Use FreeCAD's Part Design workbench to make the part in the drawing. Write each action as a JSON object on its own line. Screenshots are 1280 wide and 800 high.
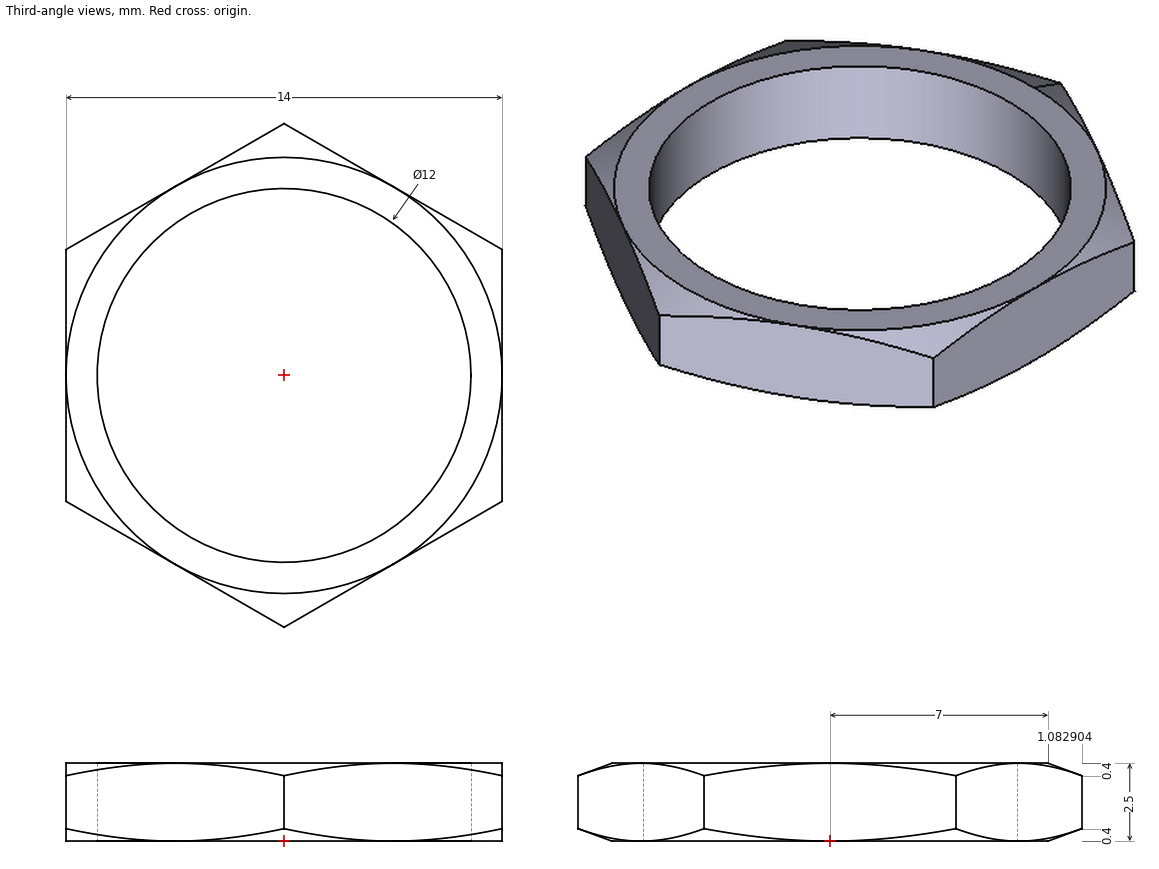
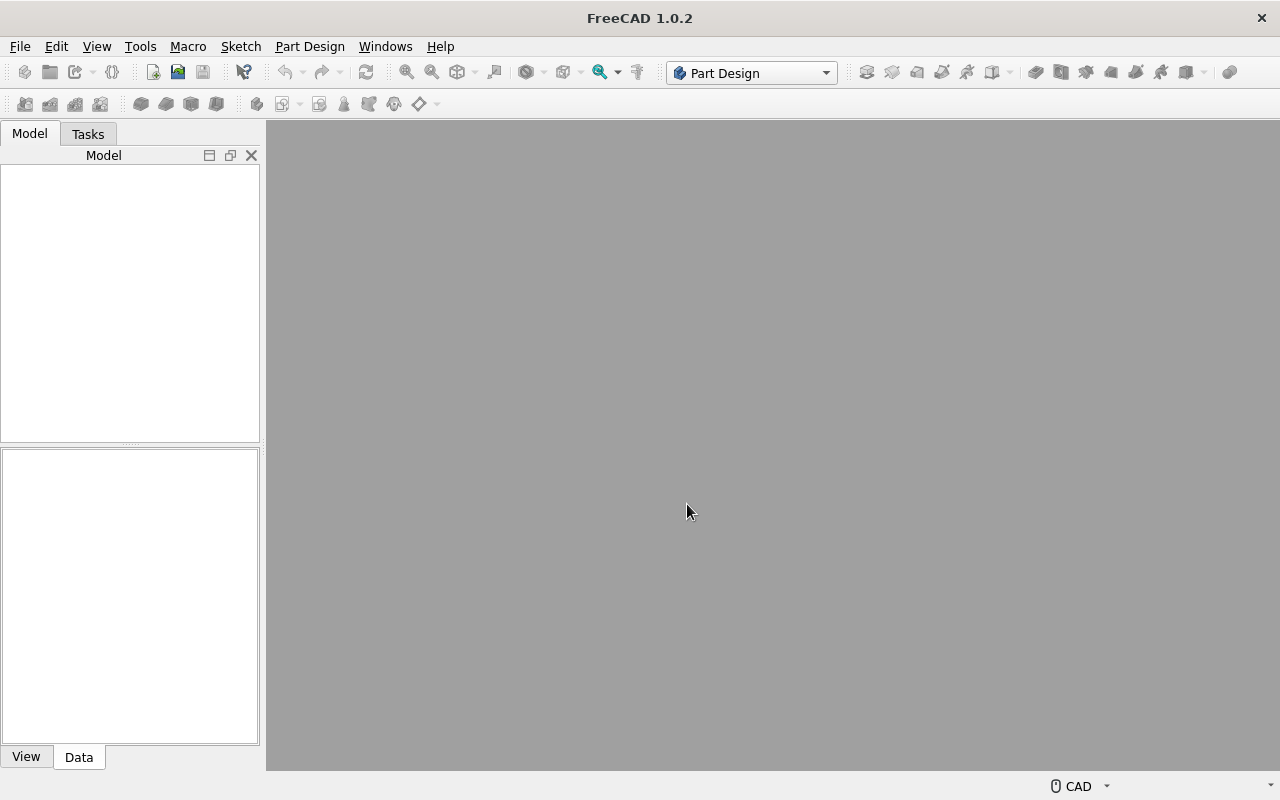
{"action": "key", "text": "ctrl+n"}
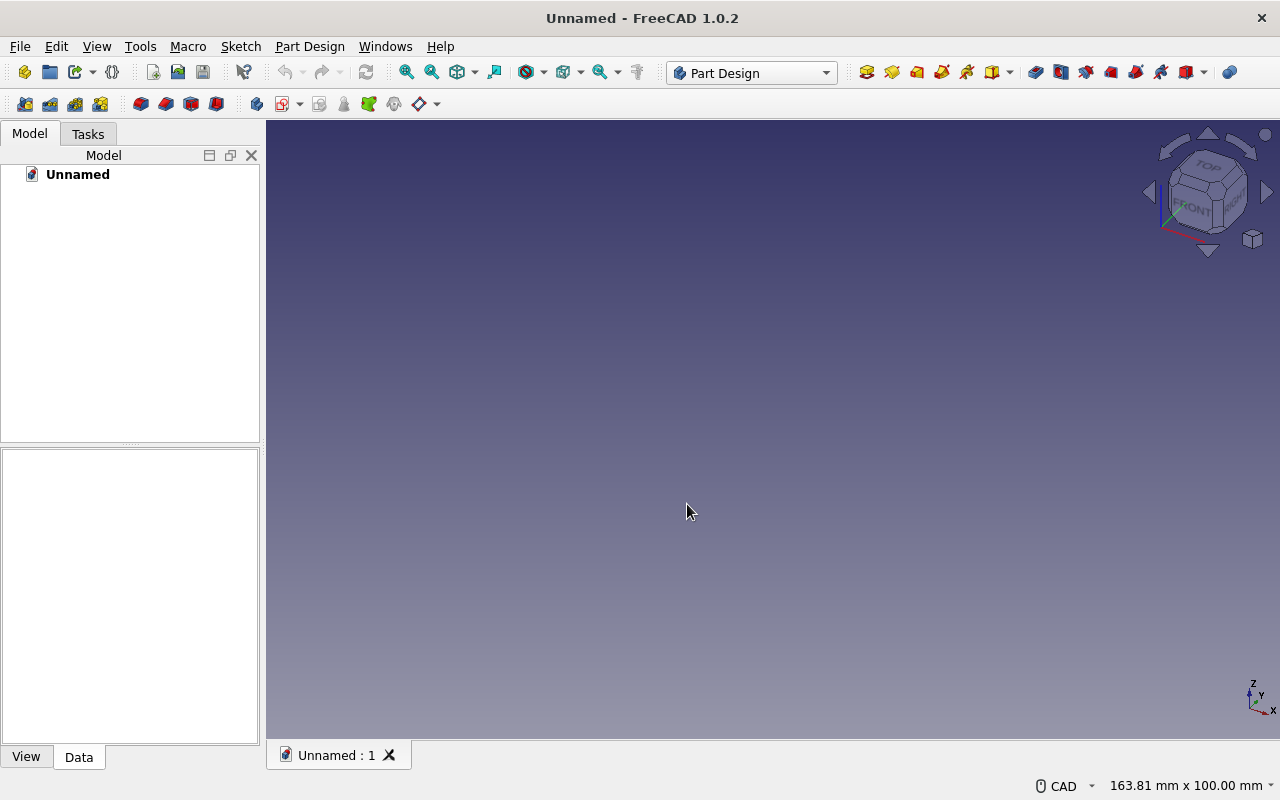
{"action": "left_click", "coordinate": [282, 104]}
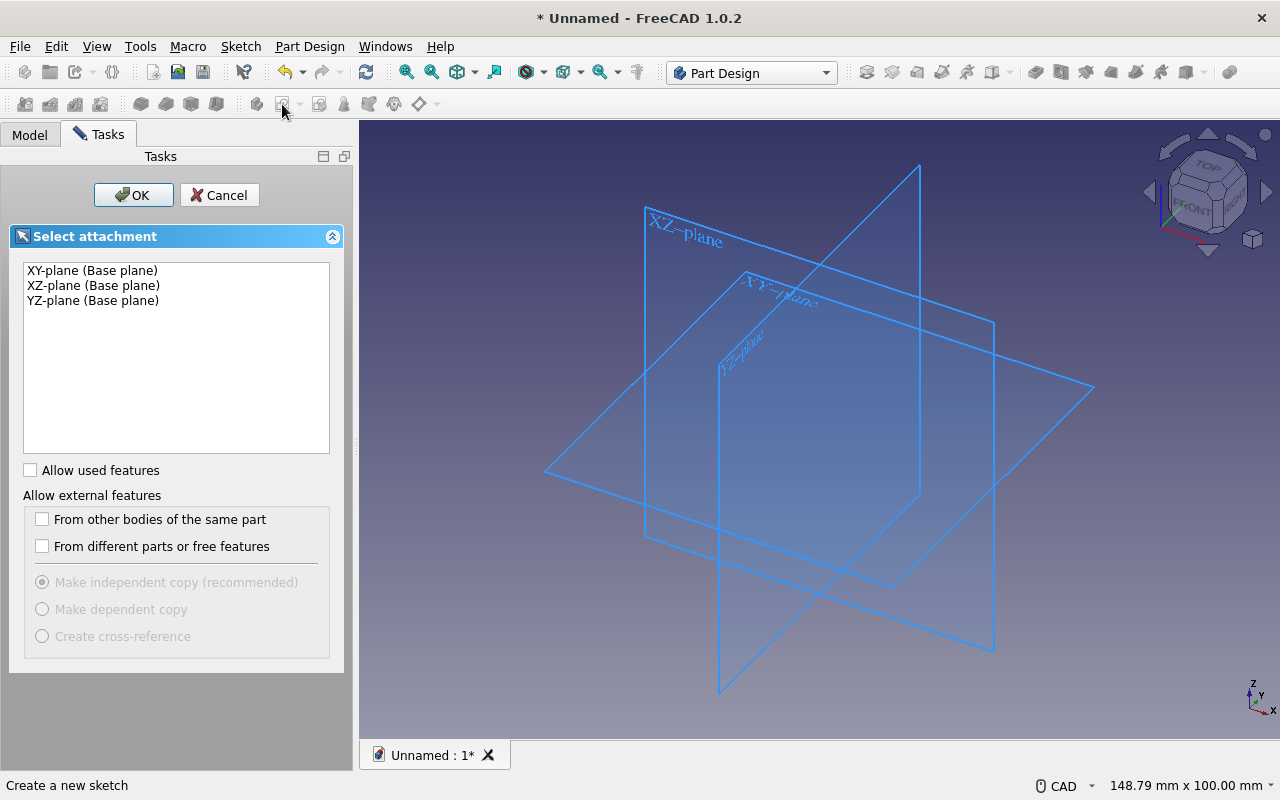
{"action": "left_click", "coordinate": [84, 270]}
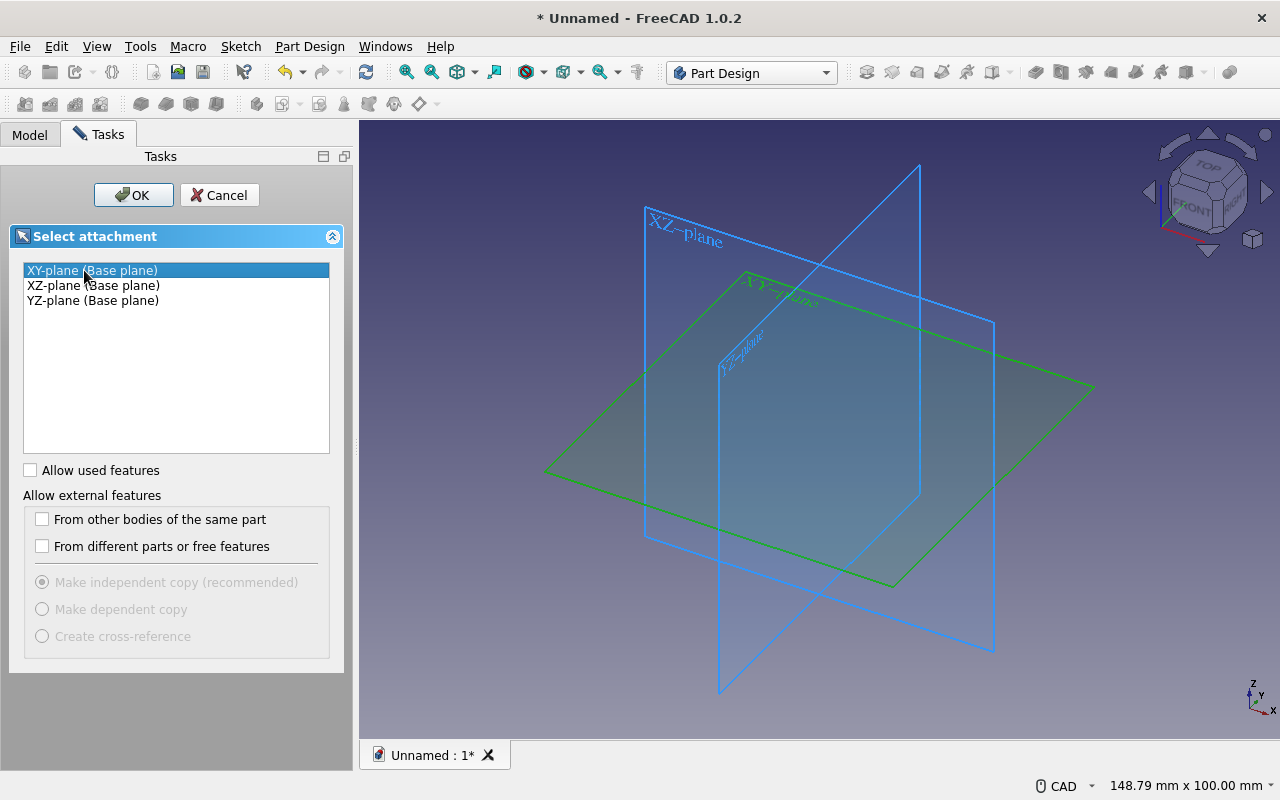
{"action": "left_click", "coordinate": [134, 195]}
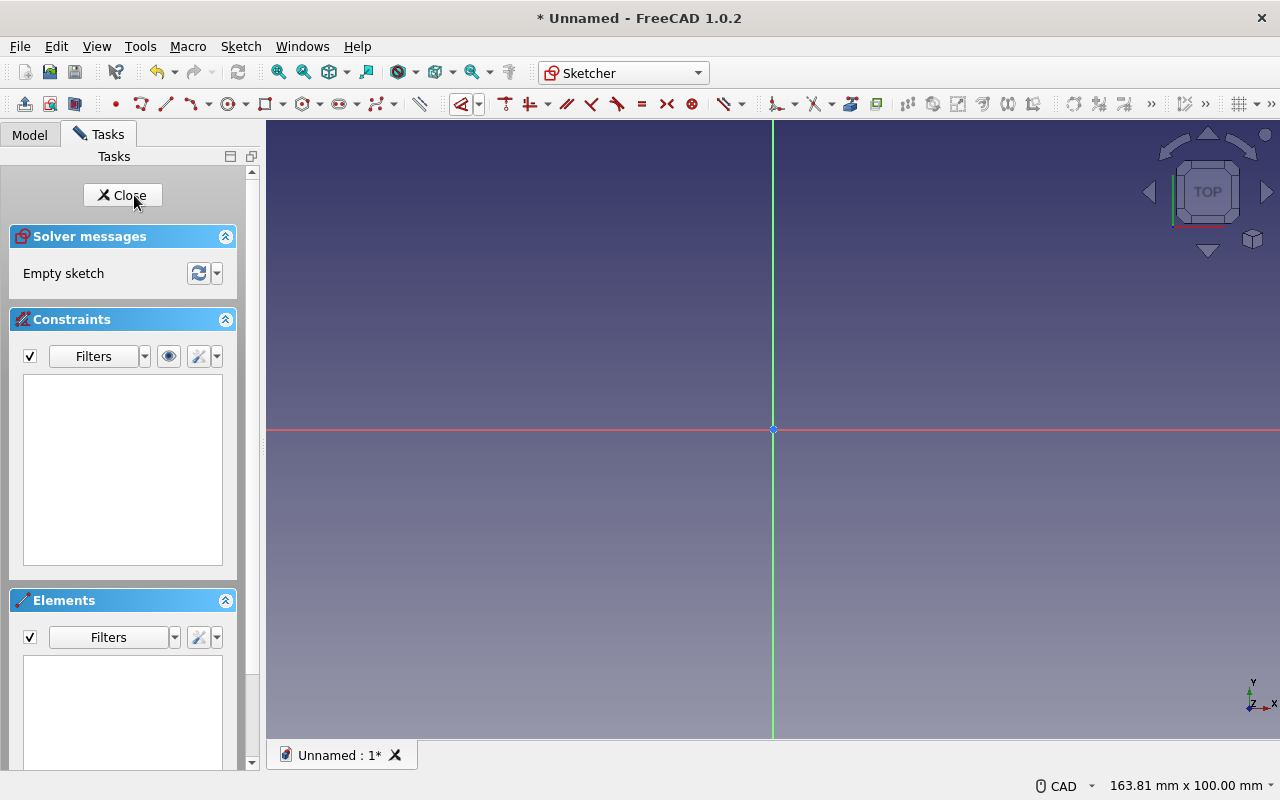
{"action": "scroll", "coordinate": [795, 430], "scroll_direction": "up", "scroll_amount": 7}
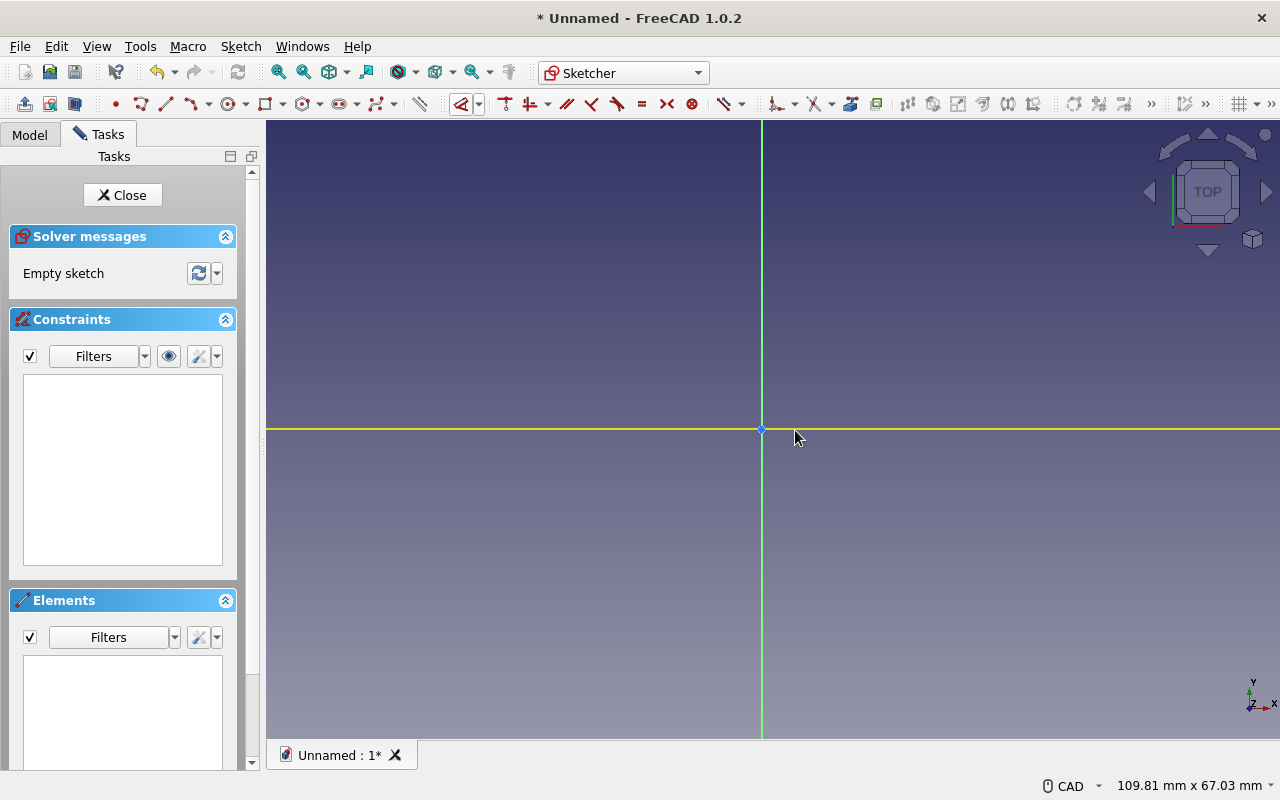
{"action": "left_click", "coordinate": [302, 104]}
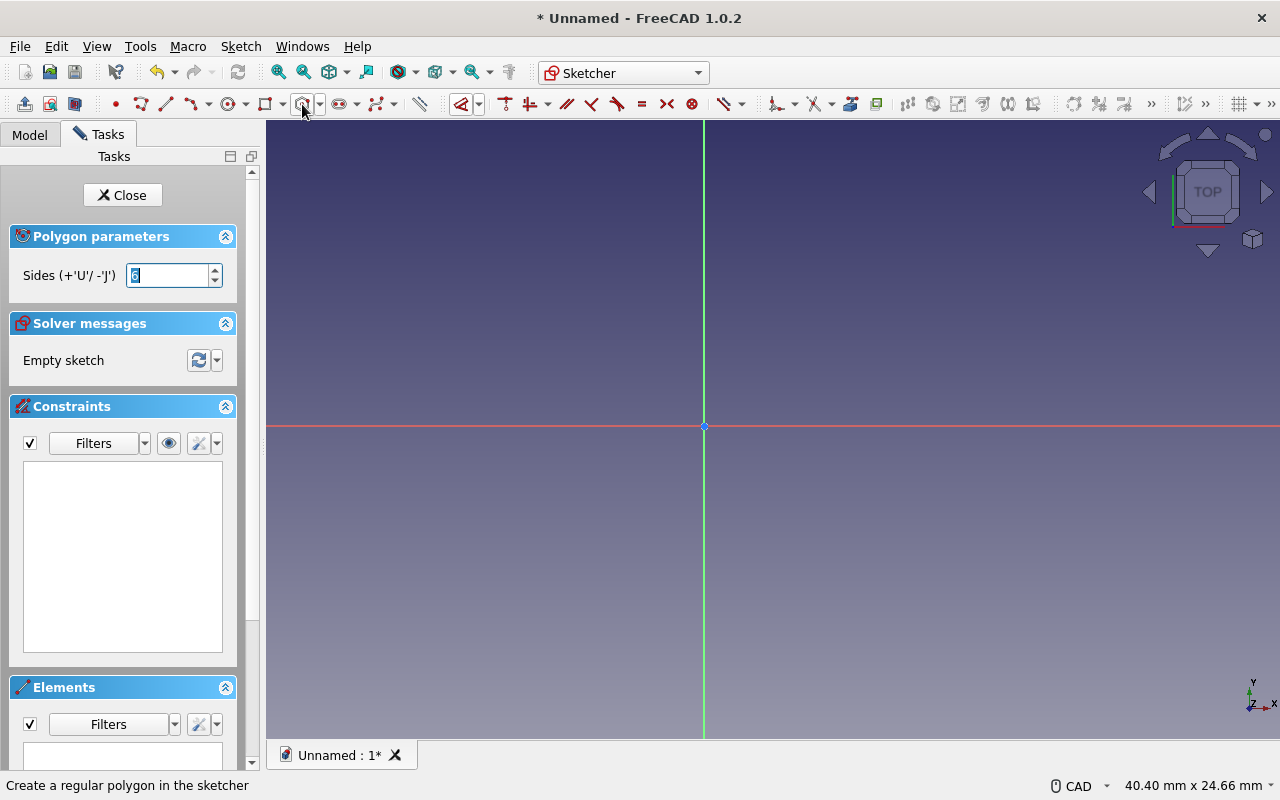
{"action": "left_click", "coordinate": [704, 426]}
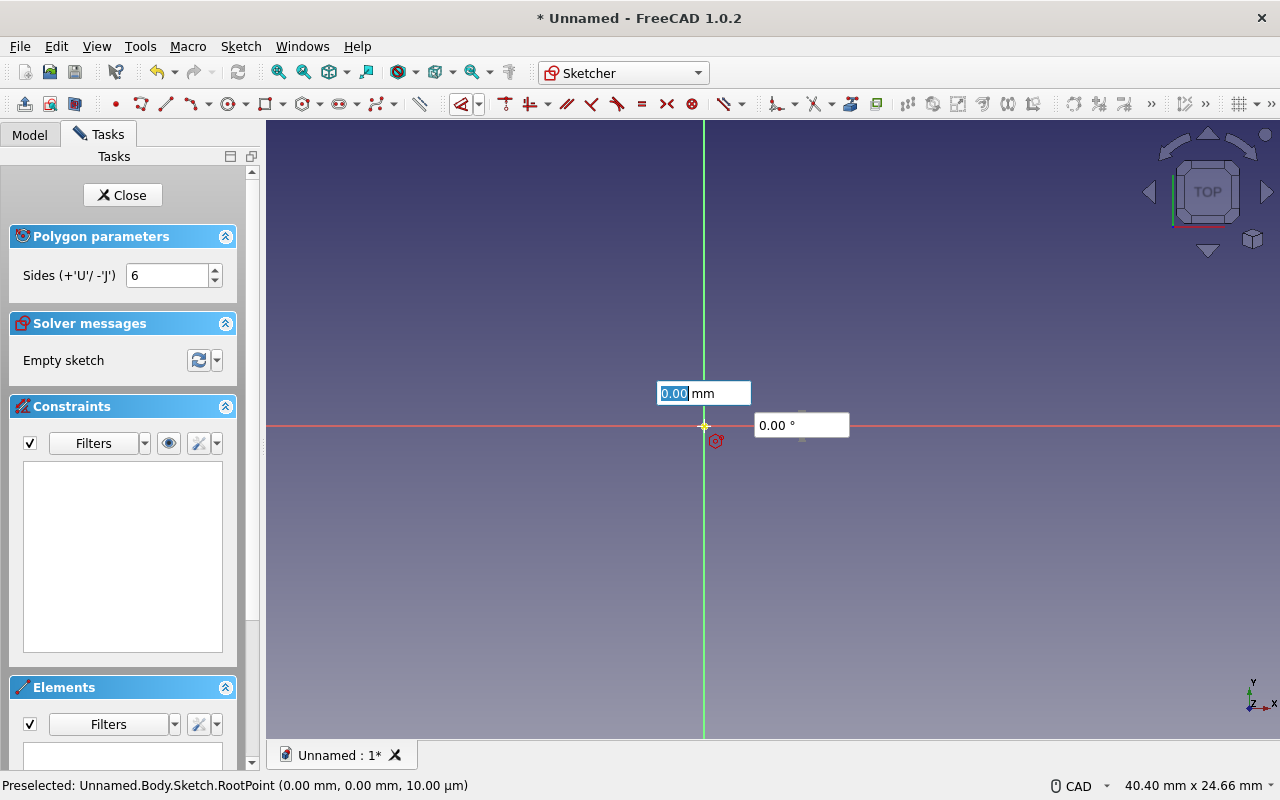
{"action": "left_click", "coordinate": [704, 224]}
{"action": "key", "text": "Escape"}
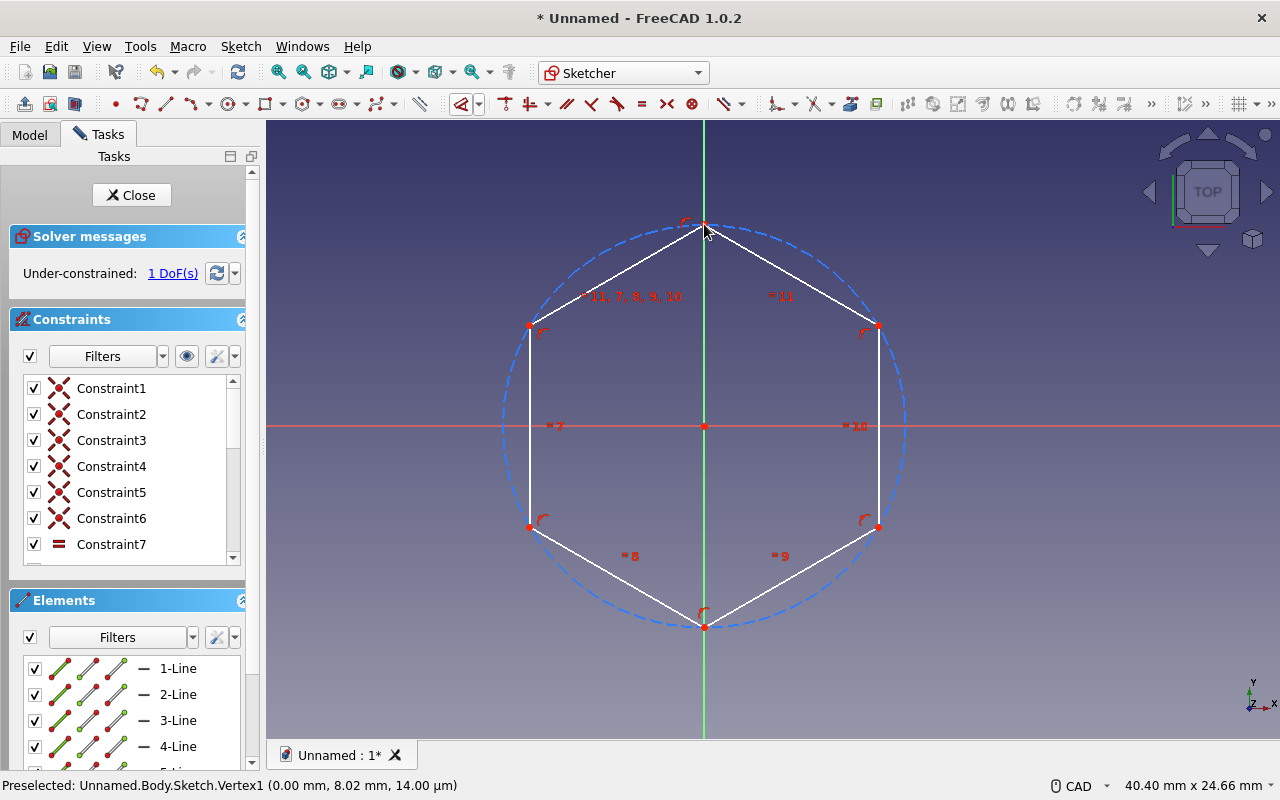
{"action": "key", "text": "g c"}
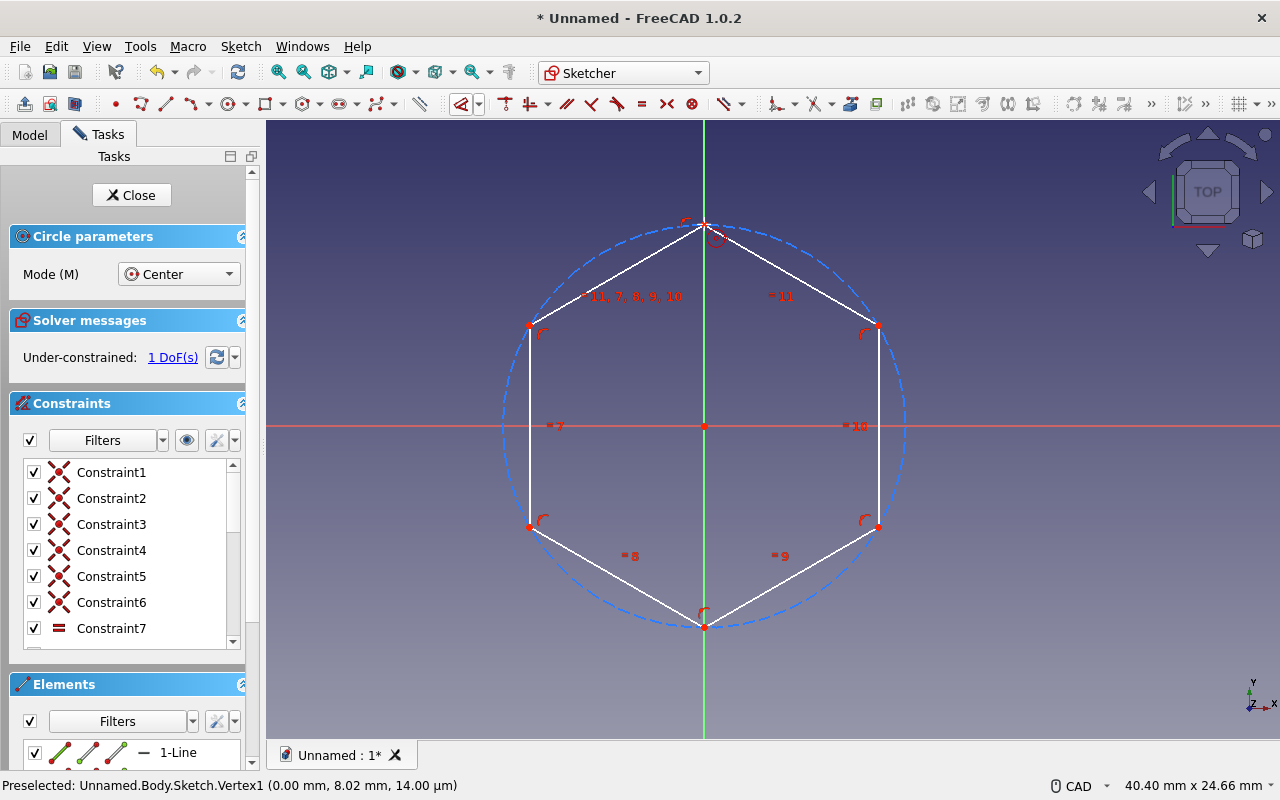
{"action": "left_click", "coordinate": [704, 426]}
{"action": "mouse_move", "coordinate": [811, 320]}